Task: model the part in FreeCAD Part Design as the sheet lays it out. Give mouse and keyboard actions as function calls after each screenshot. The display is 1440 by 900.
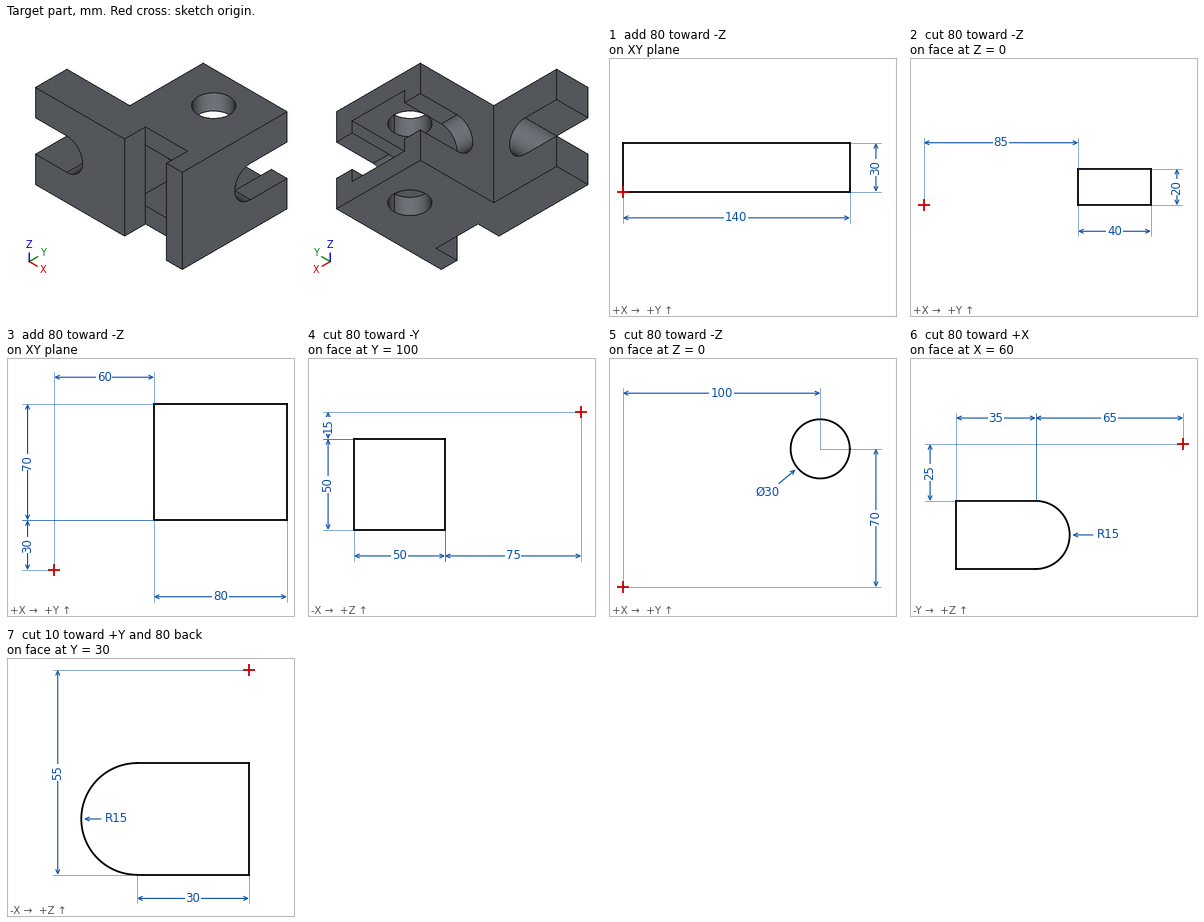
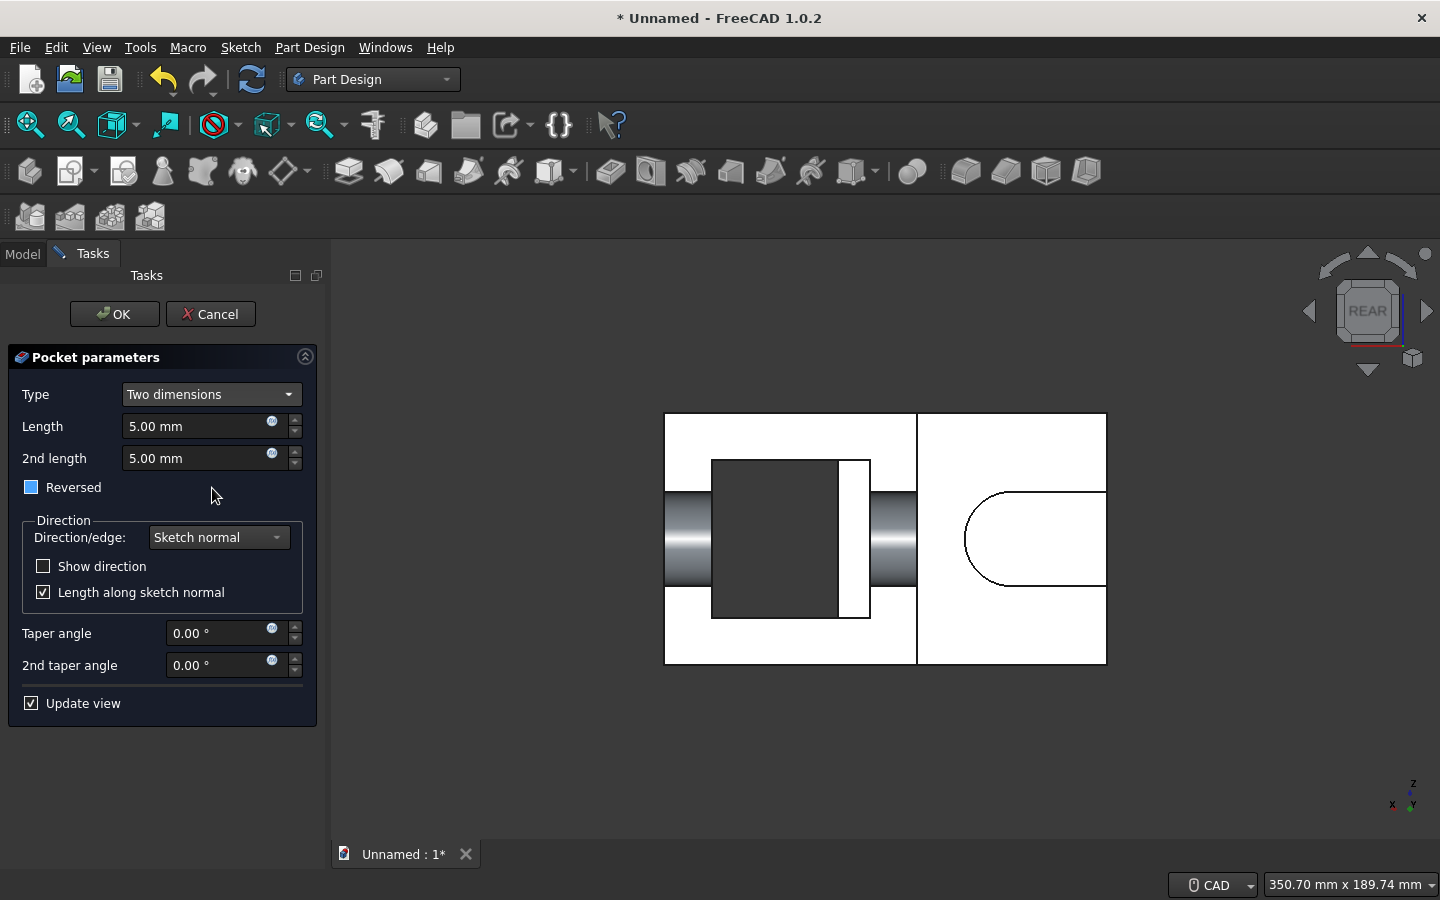
triple_click(204, 426)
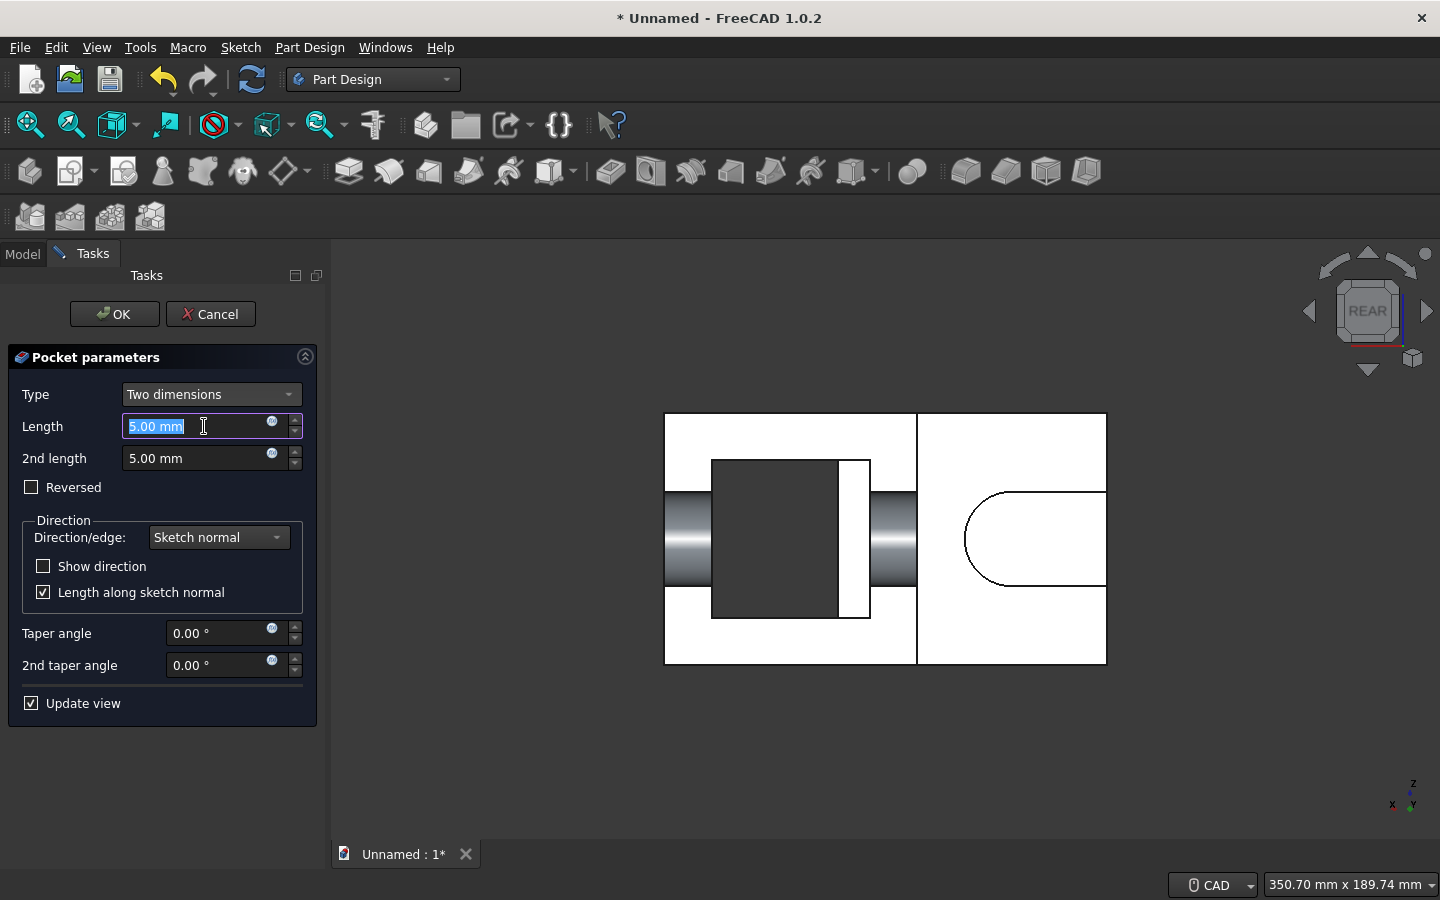
text(10)
key(Tab)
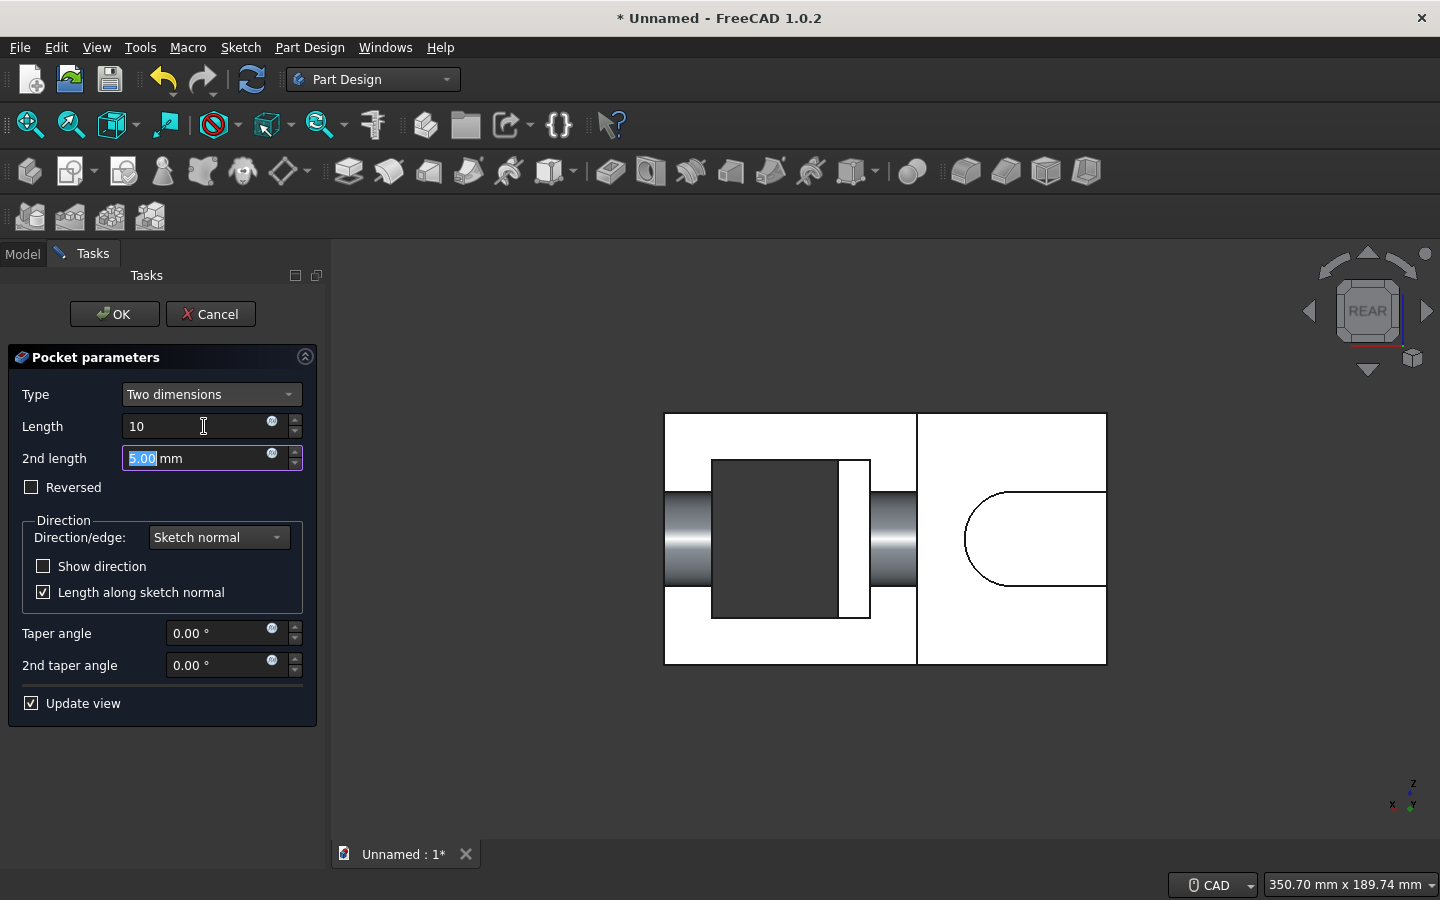
text(80)
key(Tab)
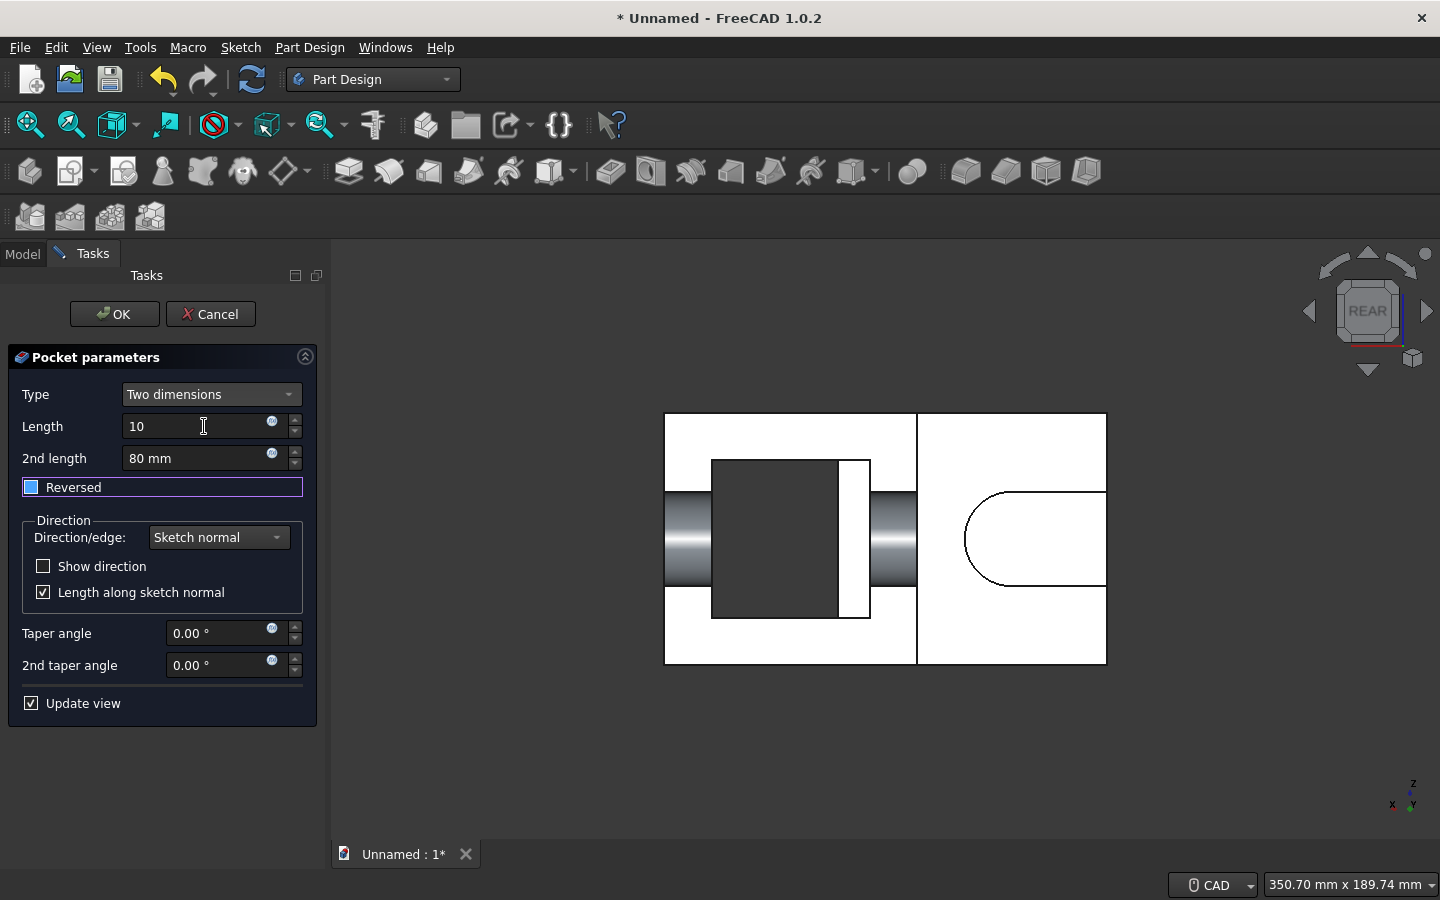
click(30, 487)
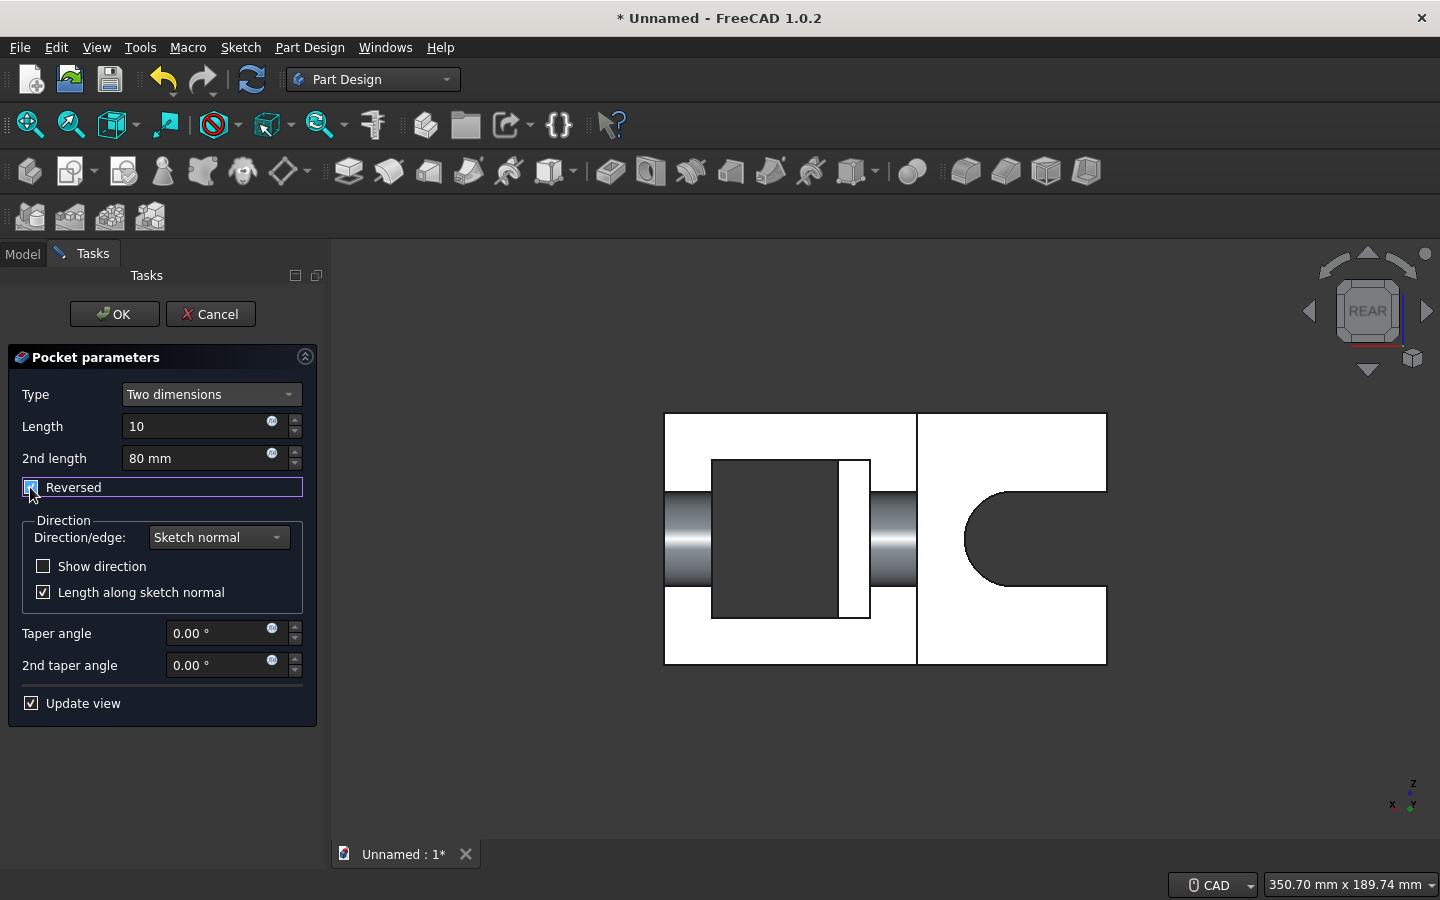
click(115, 314)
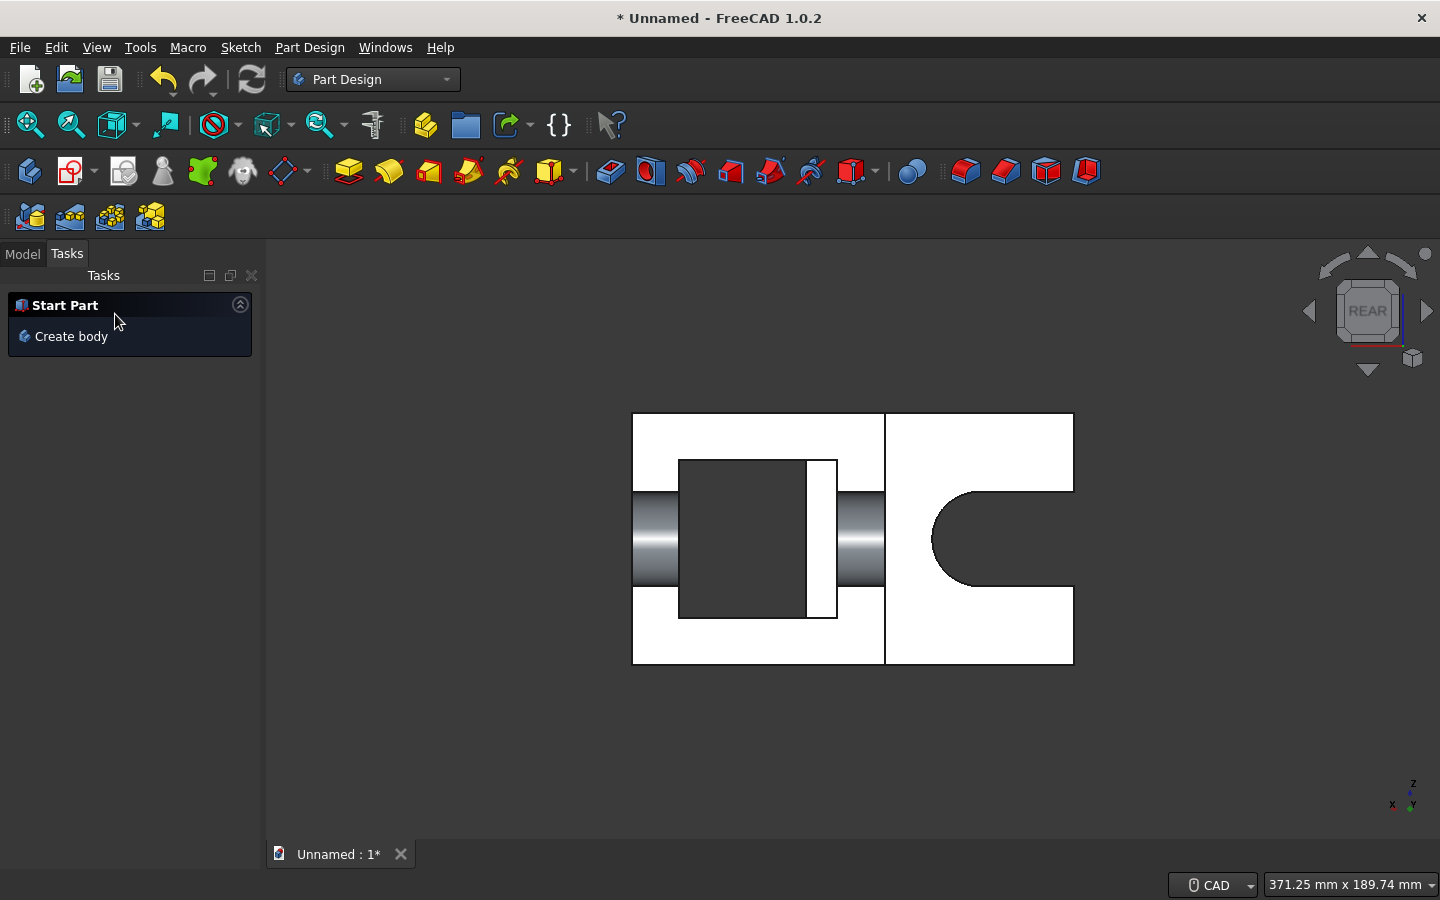
key(0)